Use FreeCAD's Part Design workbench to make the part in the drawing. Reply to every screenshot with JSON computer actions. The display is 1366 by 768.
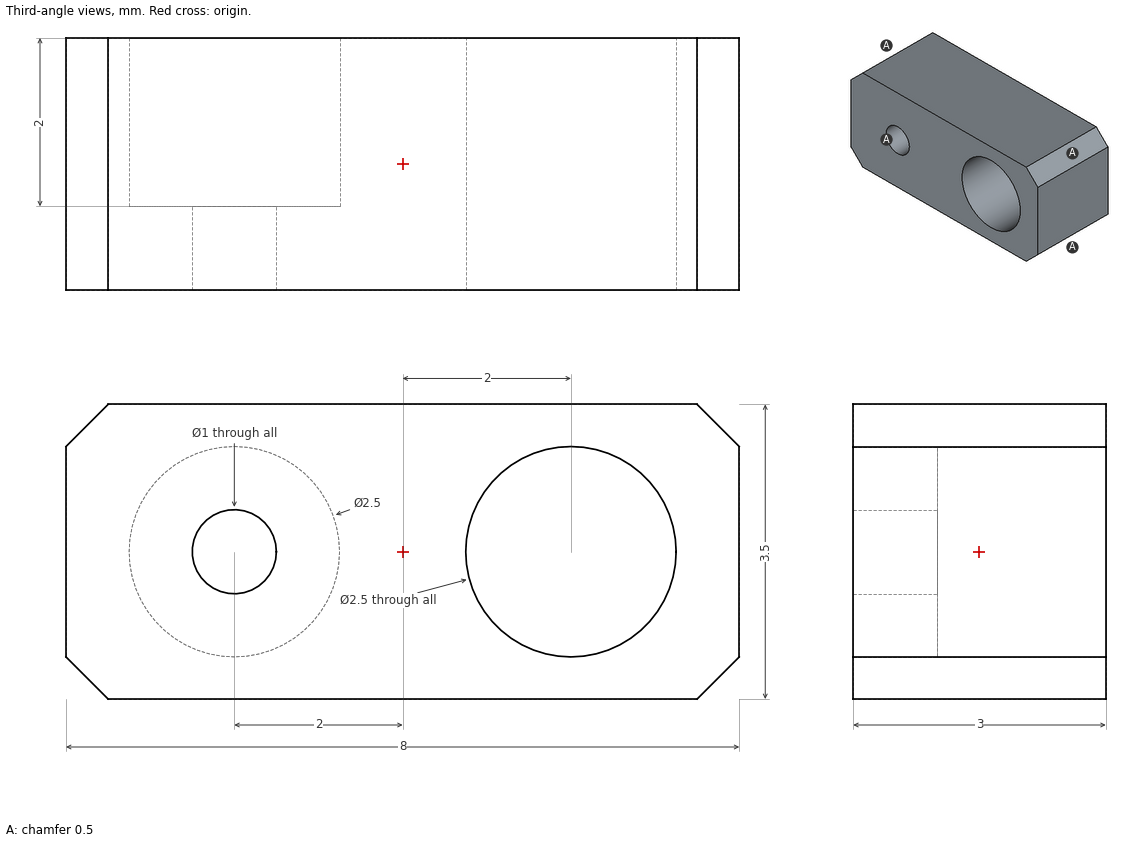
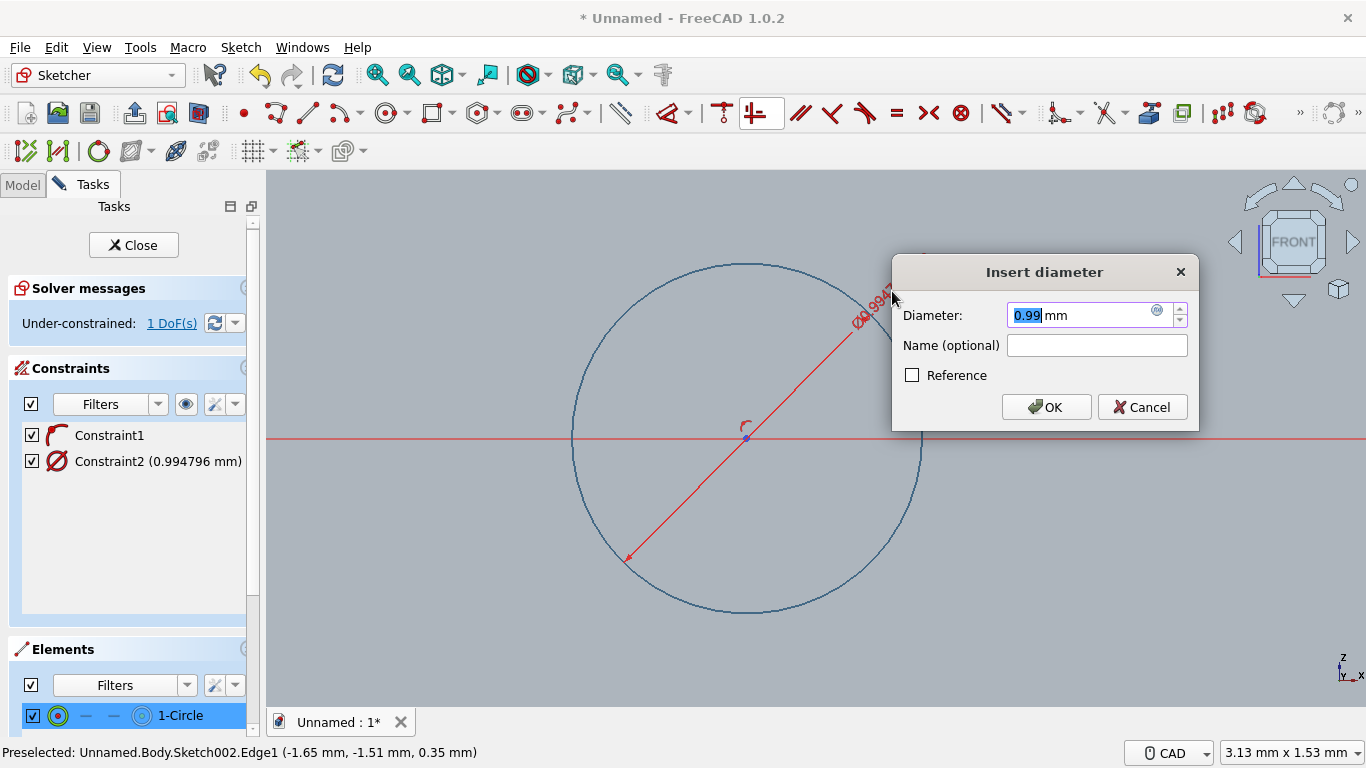
{"action": "type", "text": "1"}
{"action": "key", "text": "Return"}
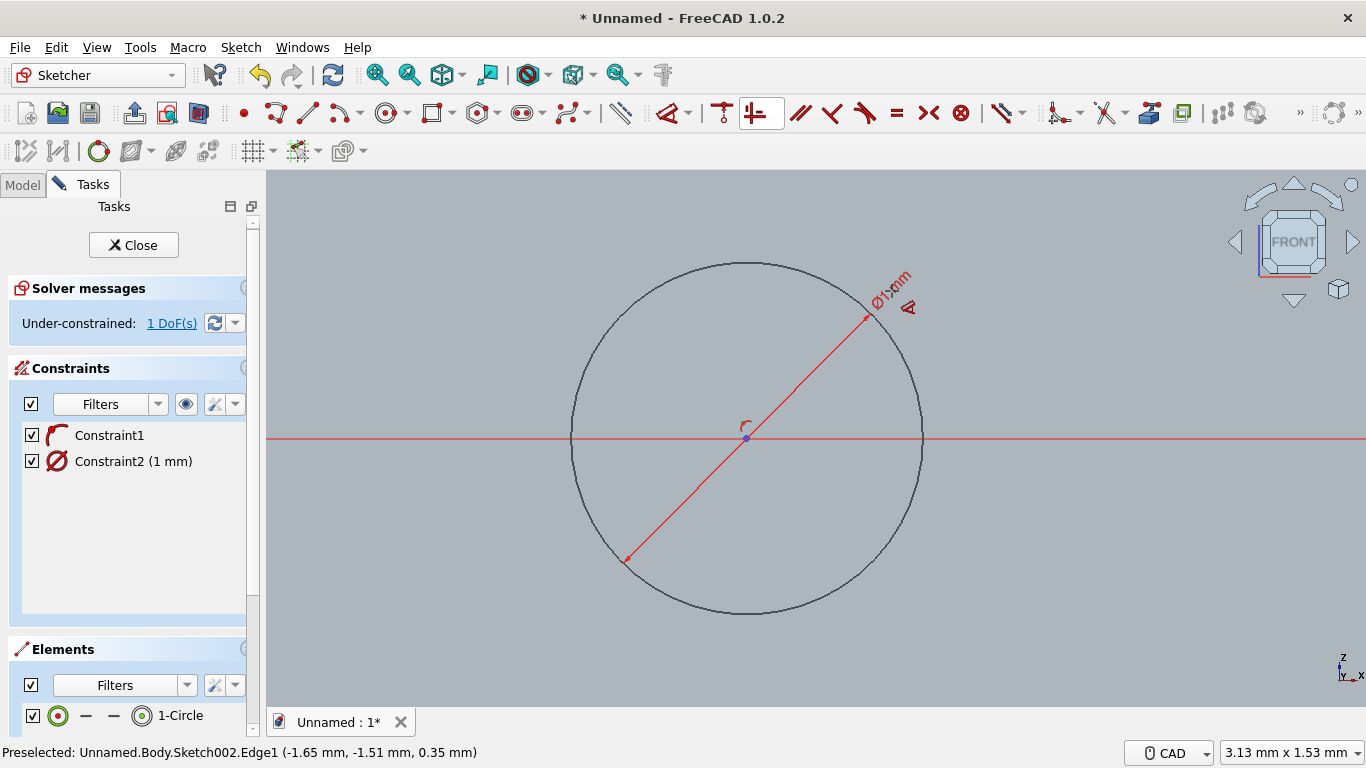
{"action": "left_click", "coordinate": [747, 438]}
{"action": "left_click", "coordinate": [974, 472]}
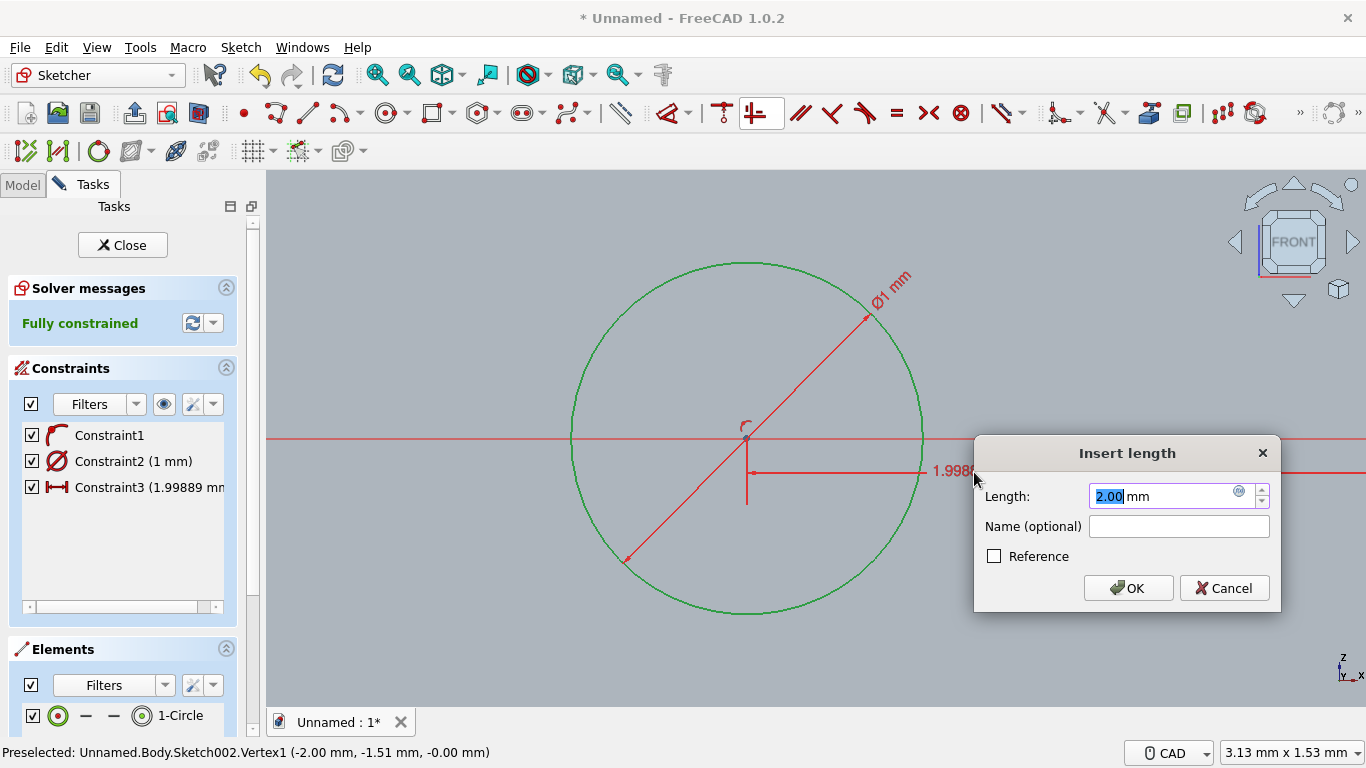
{"action": "type", "text": "2"}
{"action": "key", "text": "Return"}
{"action": "key", "text": "Escape"}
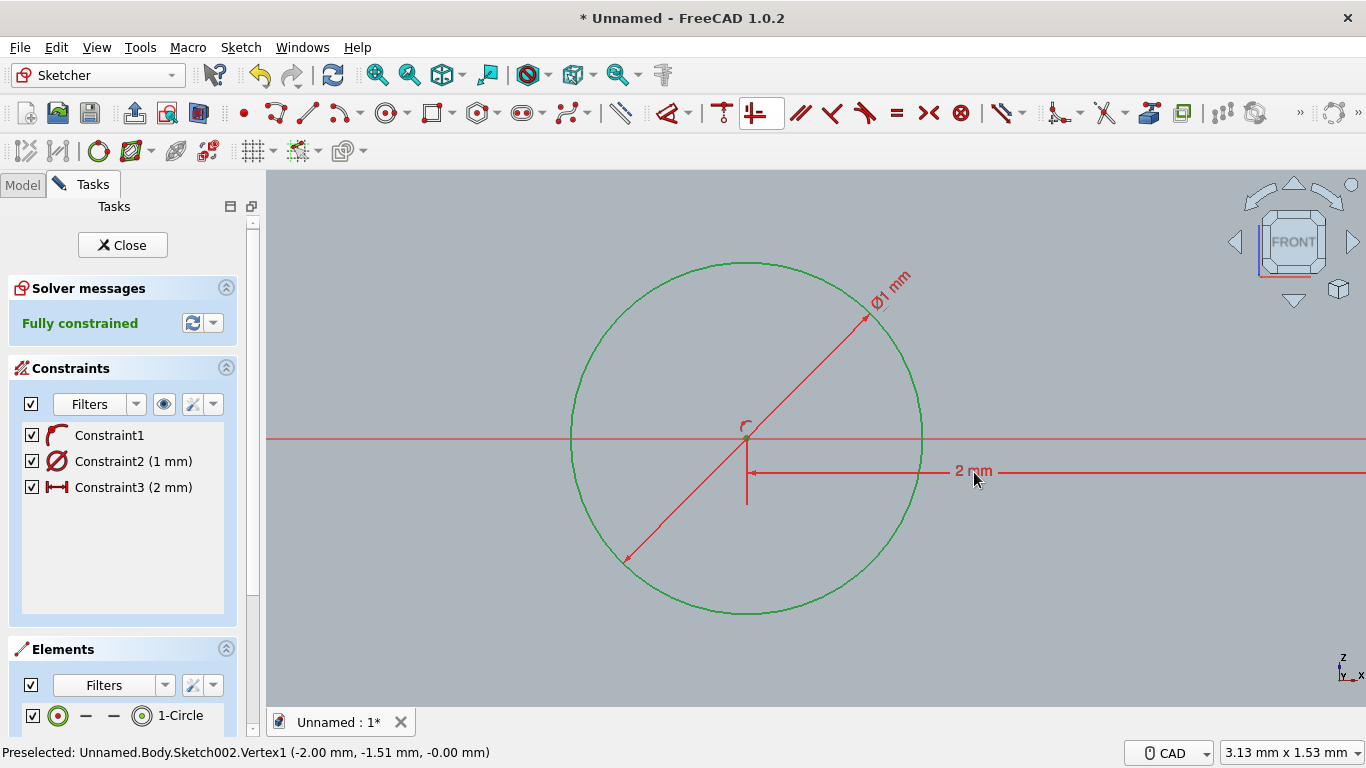
{"action": "left_click", "coordinate": [123, 245]}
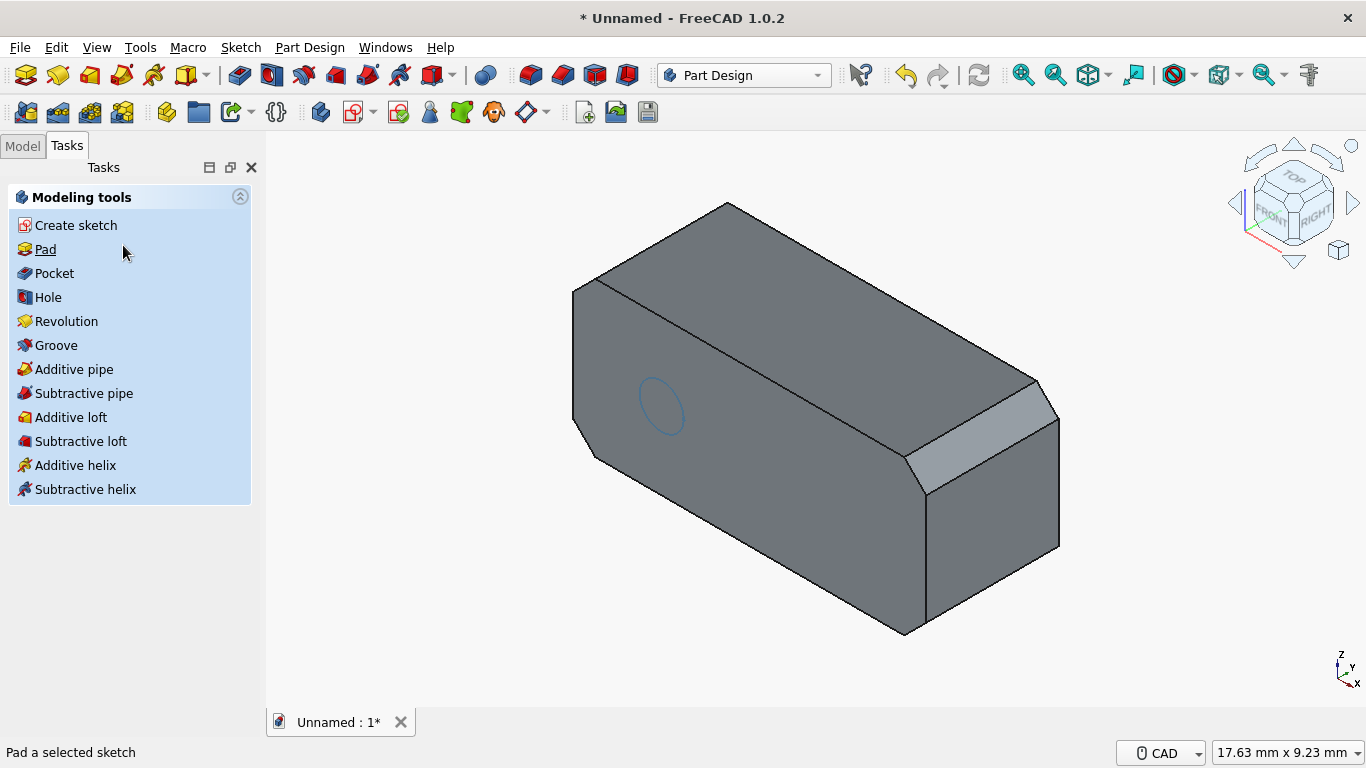
{"action": "left_click", "coordinate": [272, 76]}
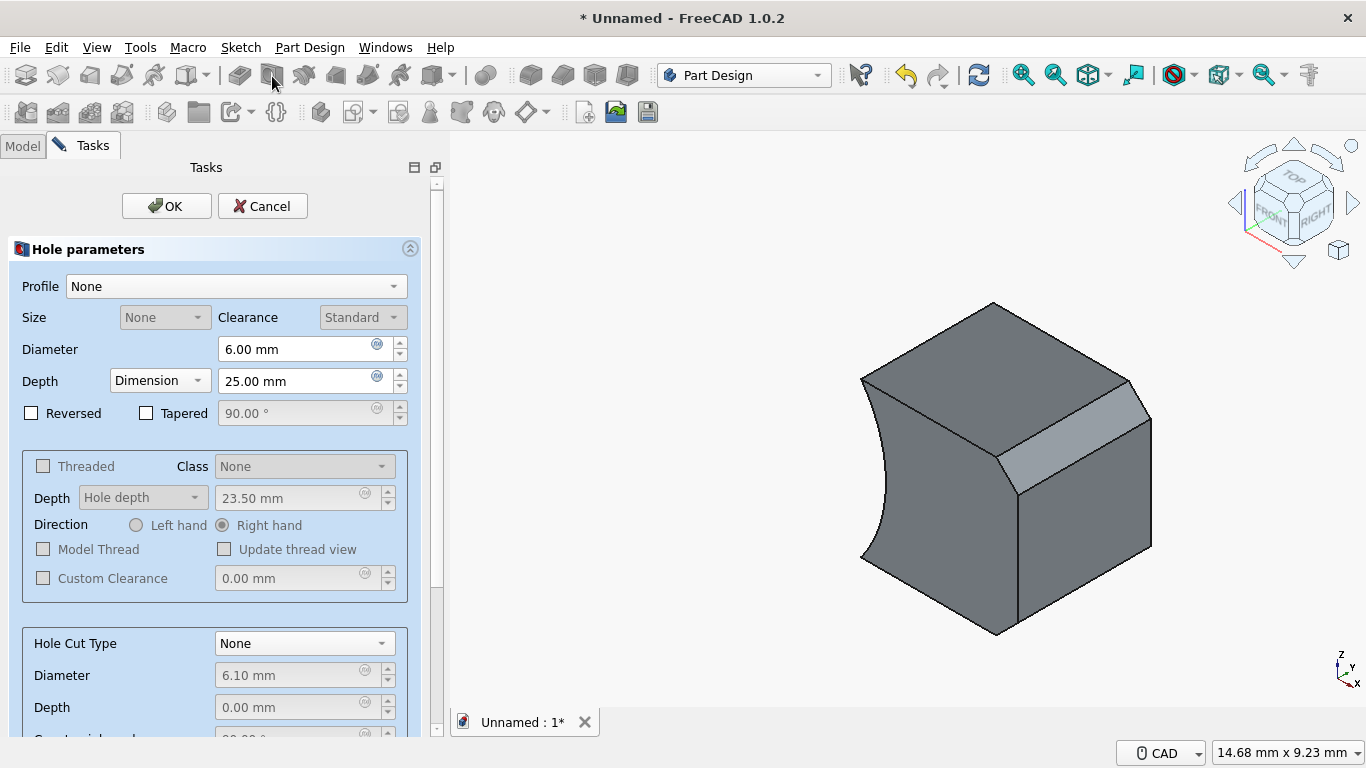
{"action": "triple_click", "coordinate": [305, 349]}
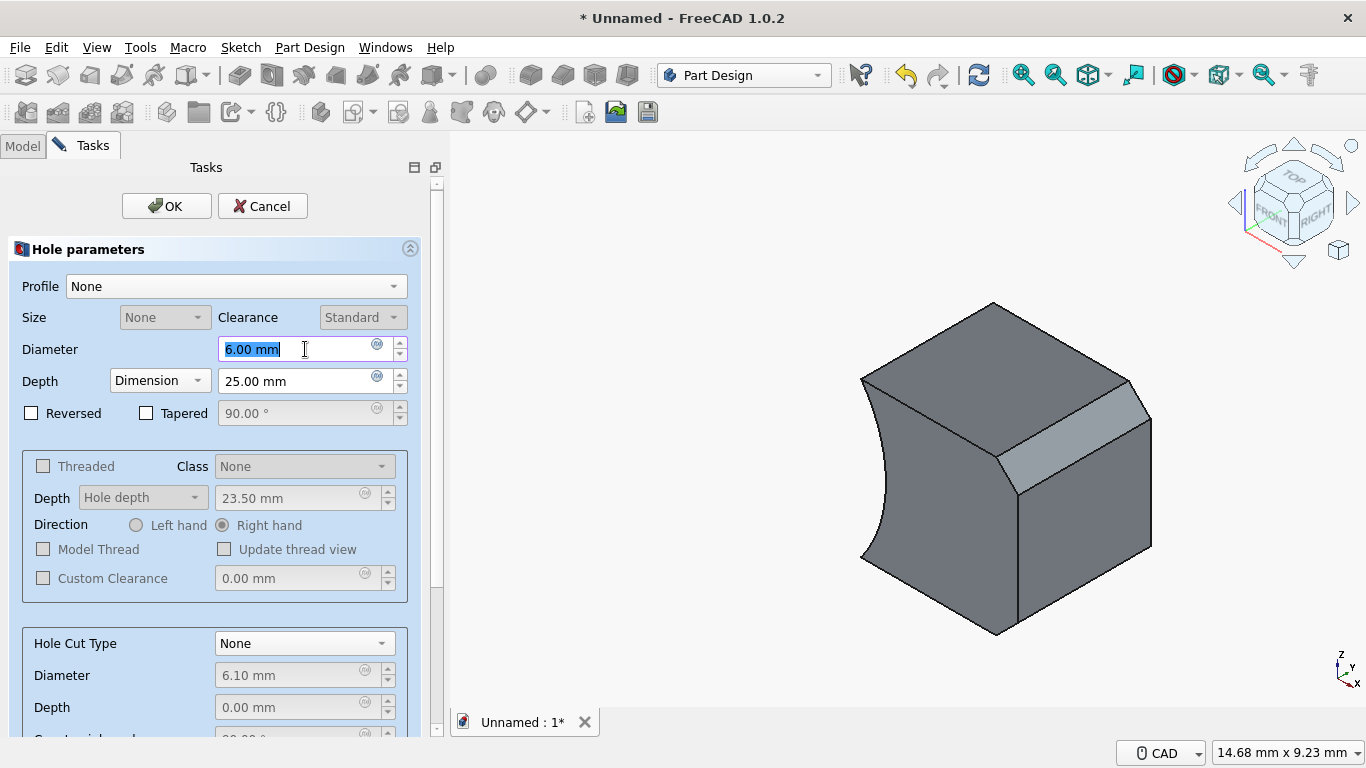
{"action": "type", "text": "1"}
{"action": "key", "text": "Tab"}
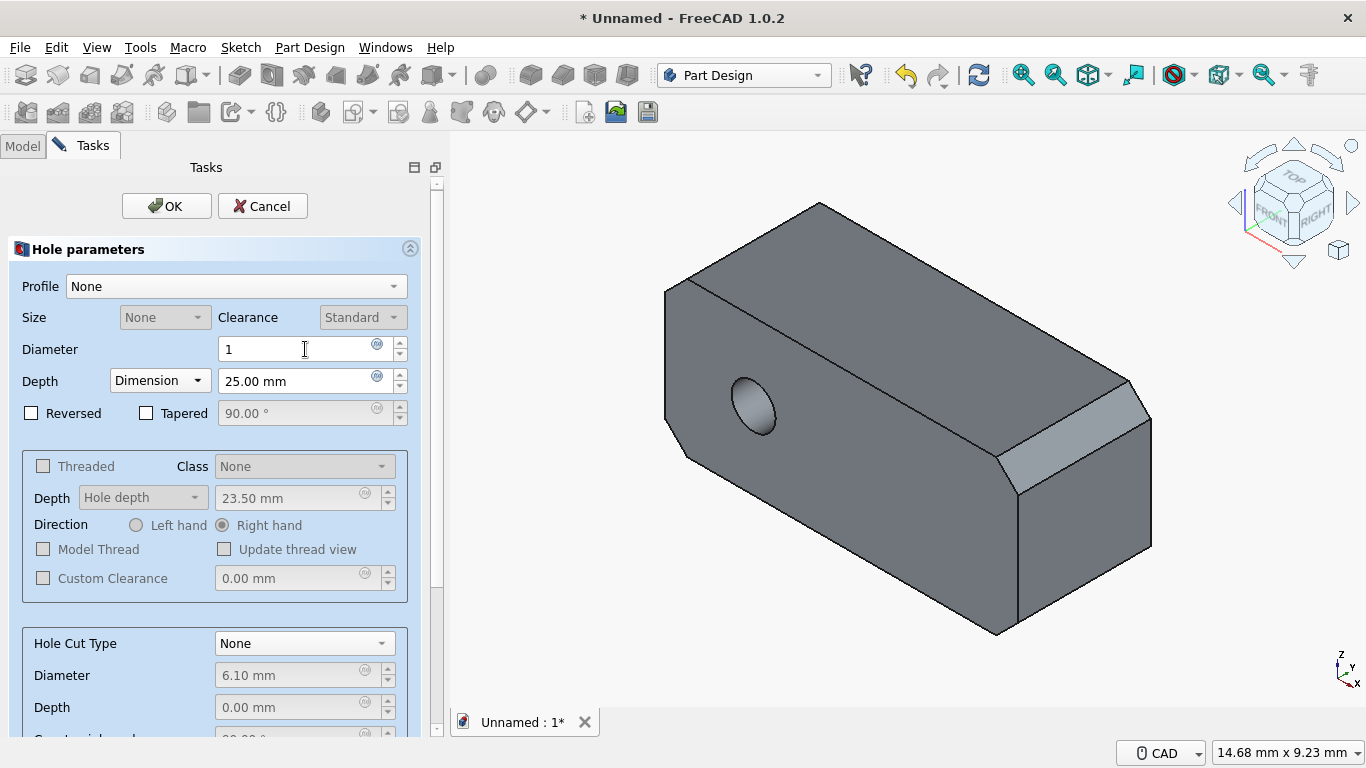
{"action": "left_click", "coordinate": [161, 380]}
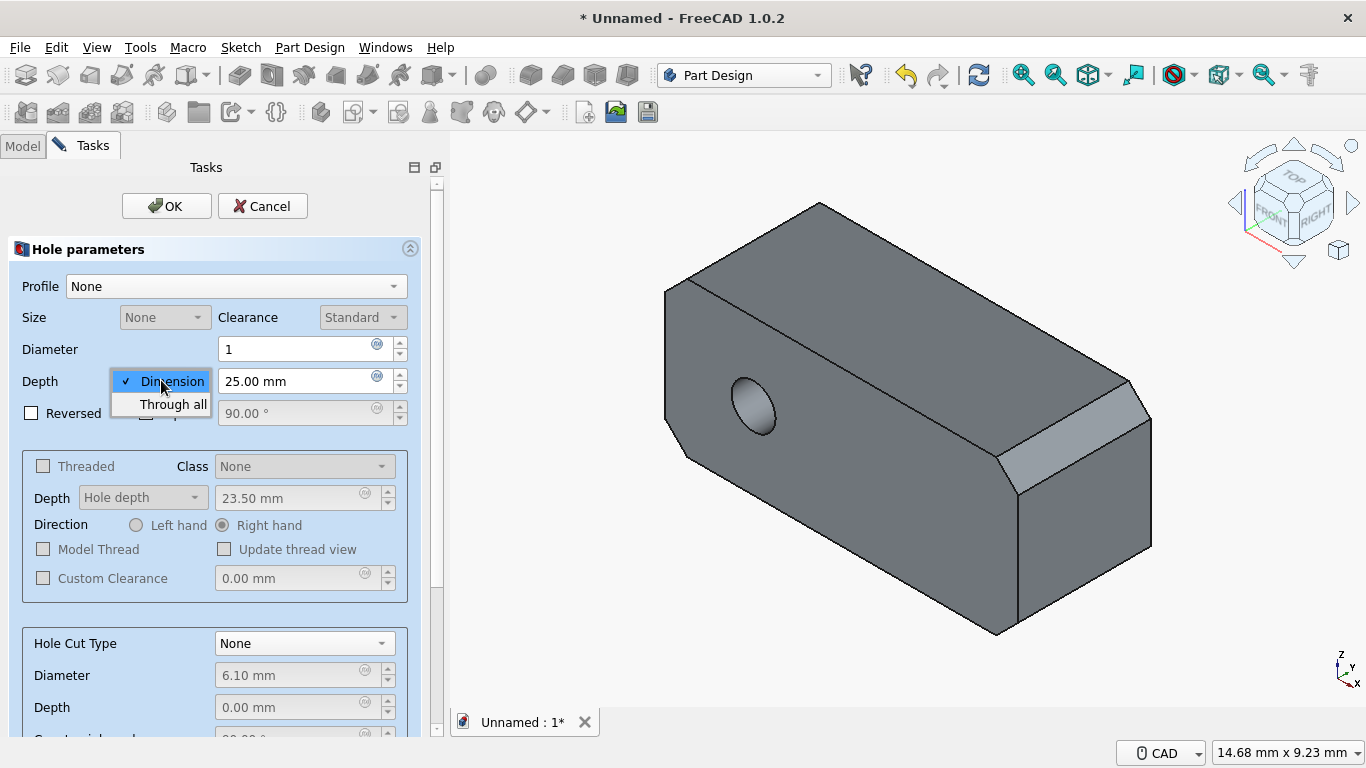
{"action": "left_click", "coordinate": [160, 404]}